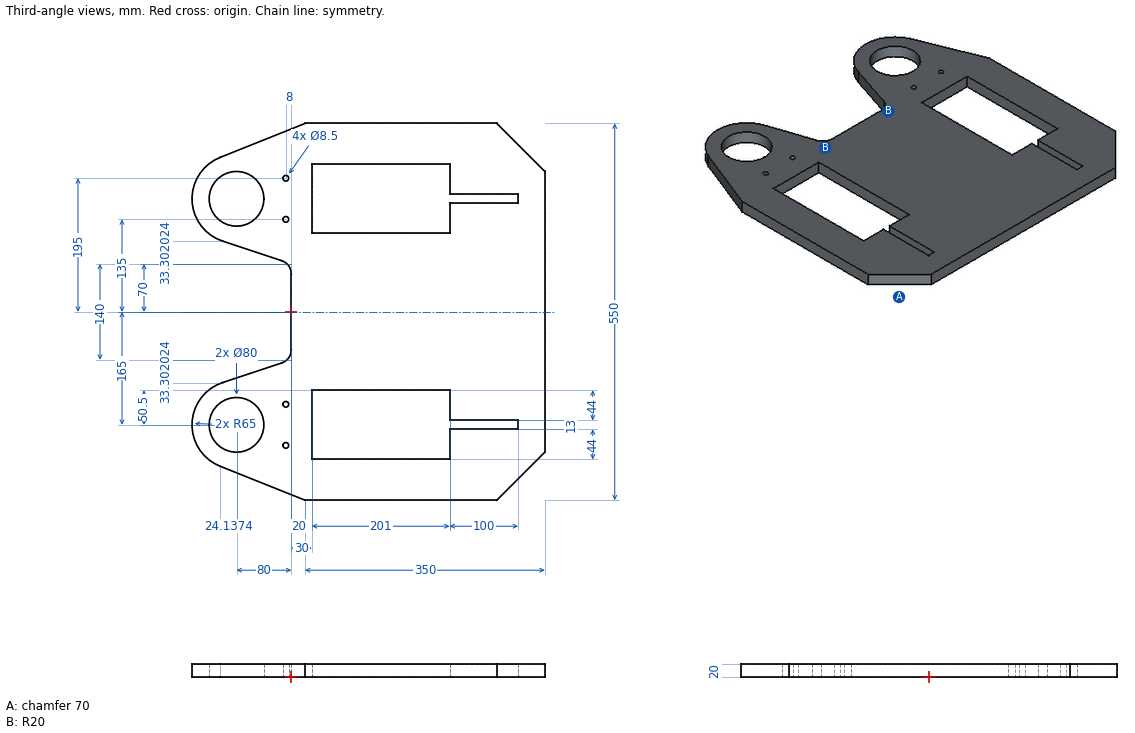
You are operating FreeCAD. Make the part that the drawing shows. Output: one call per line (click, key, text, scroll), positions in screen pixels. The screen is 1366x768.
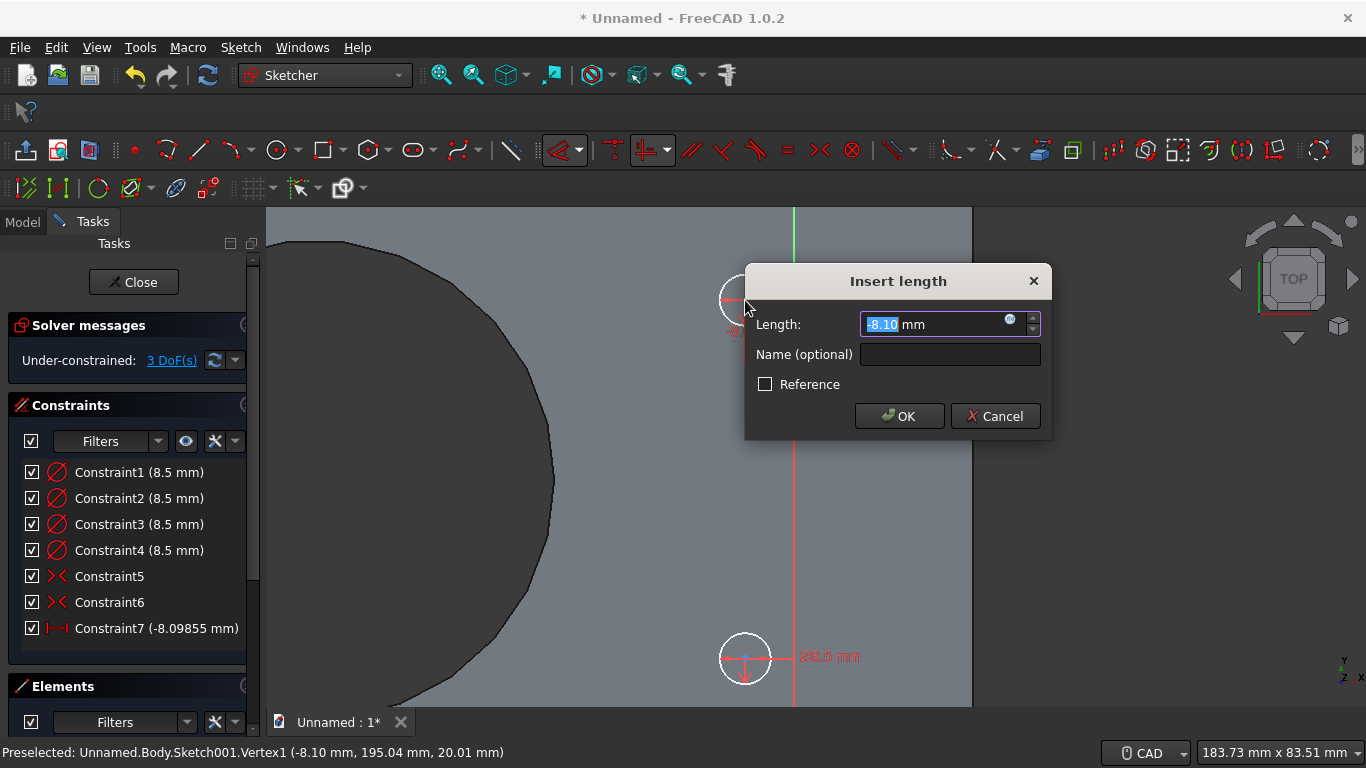
text(-8)
key(Return)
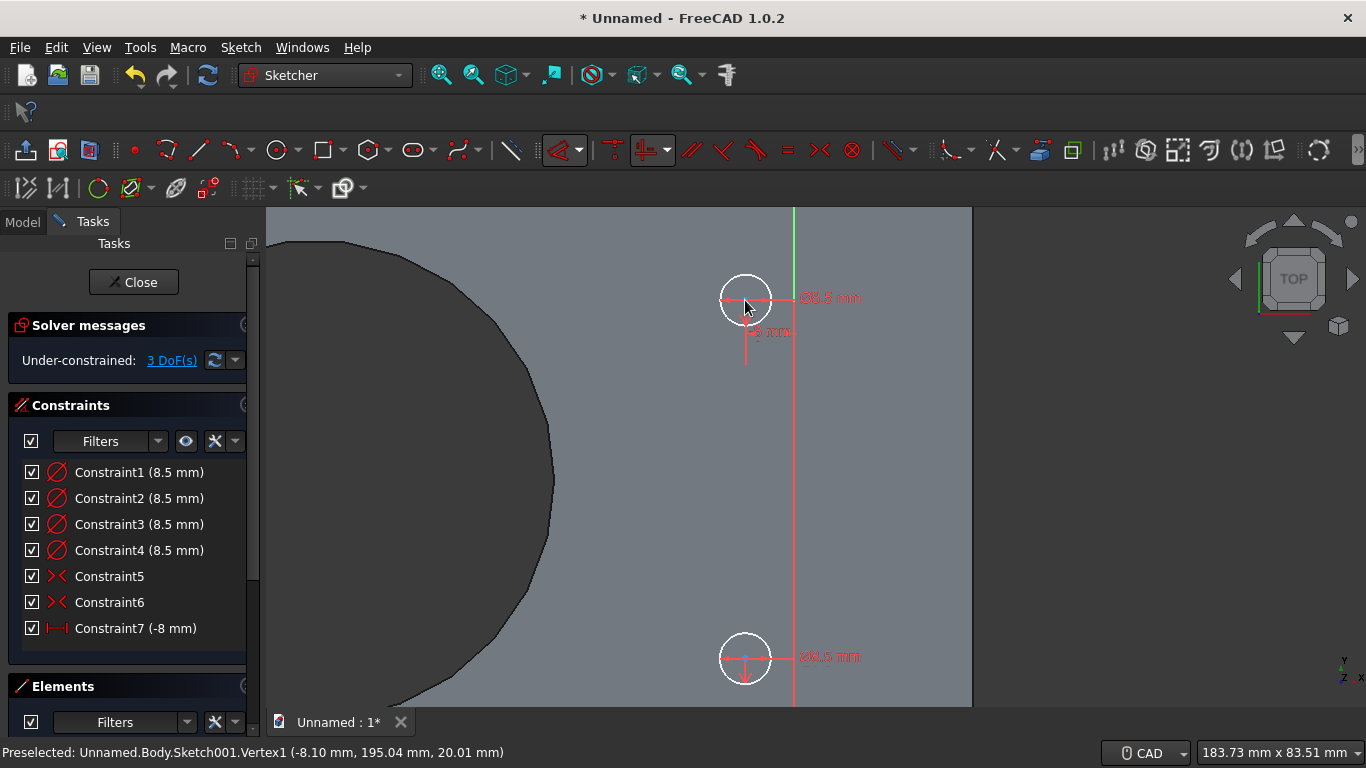
click(745, 659)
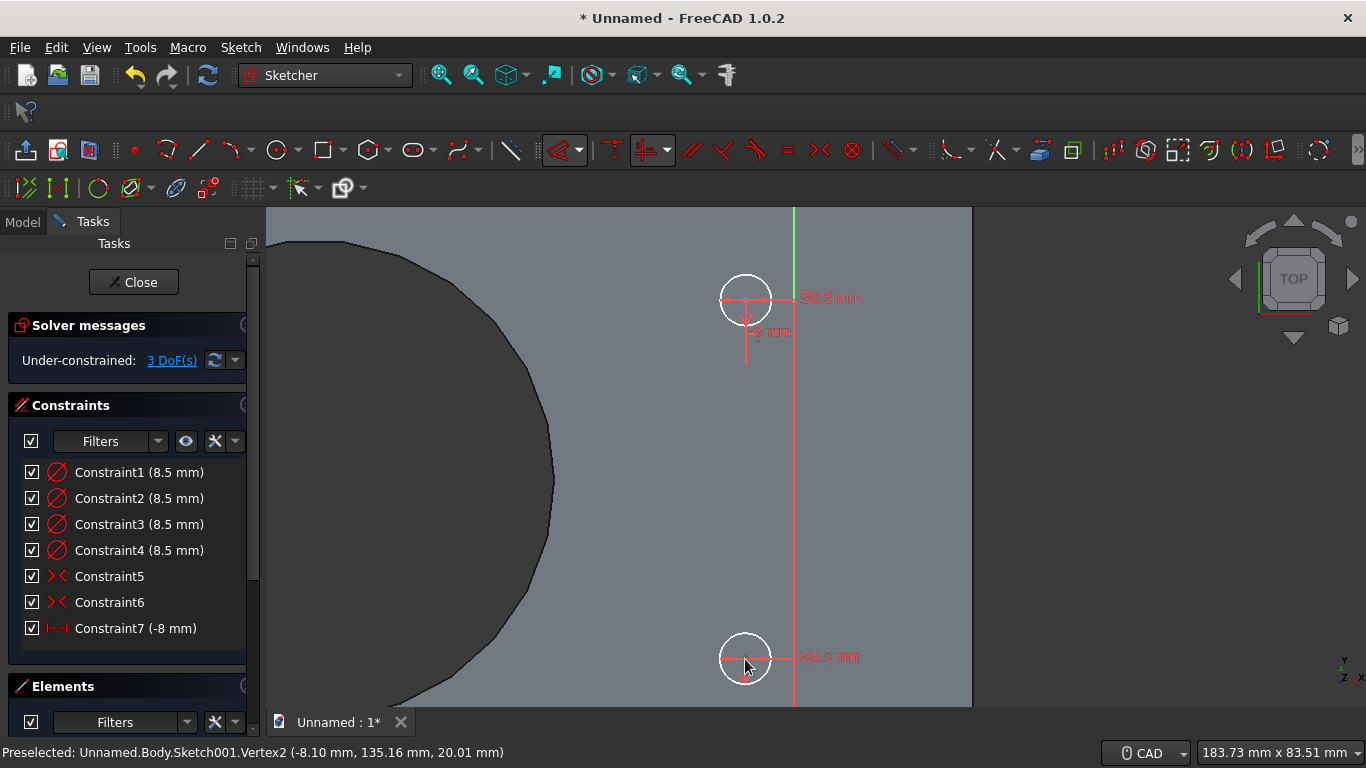
key(l)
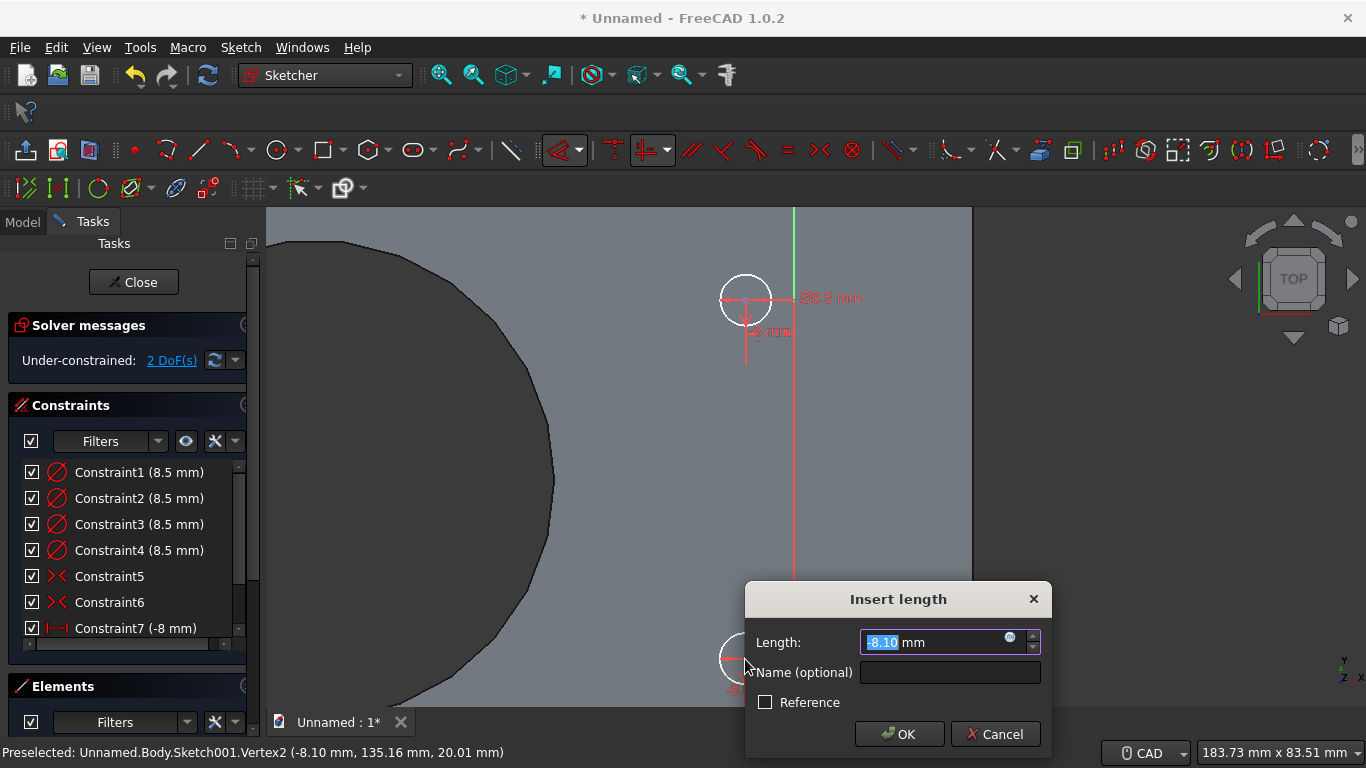
text(-8)
key(Return)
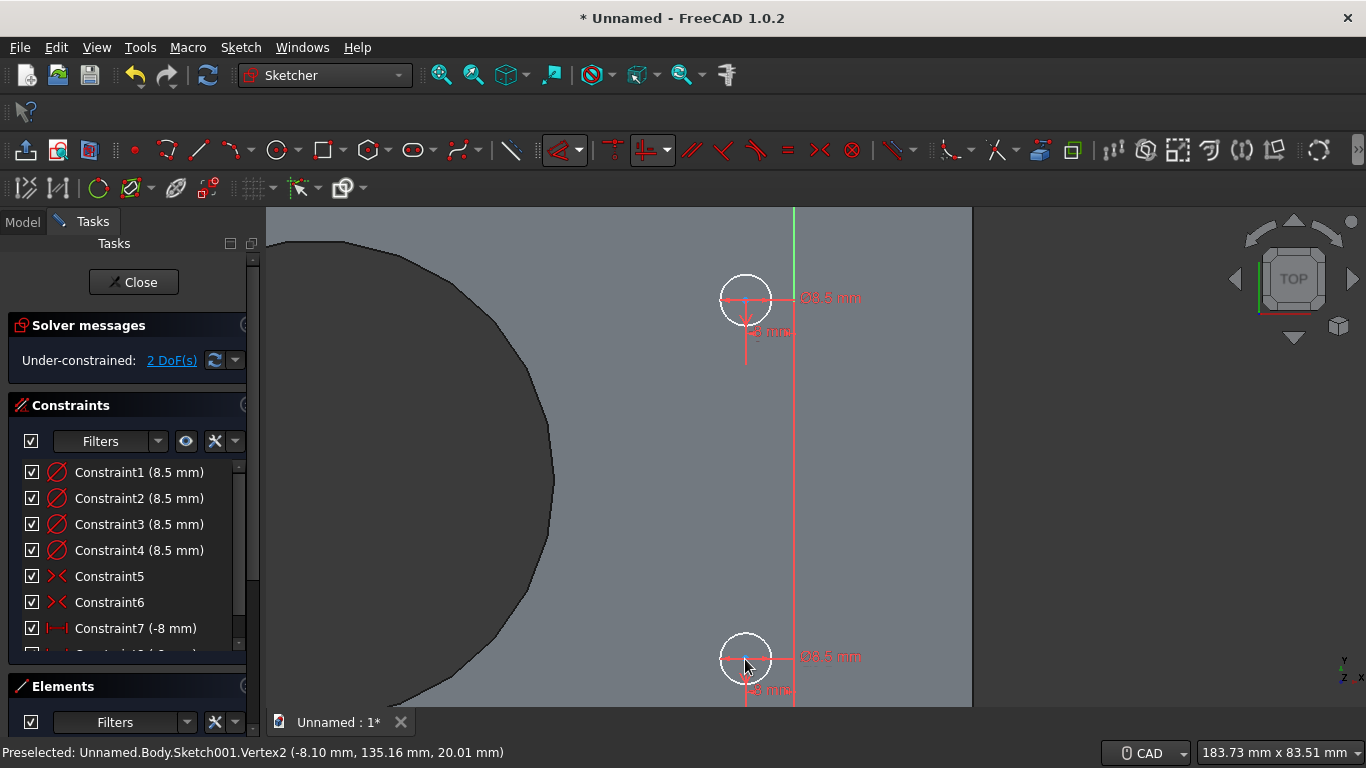
scroll(746, 299, down, 10)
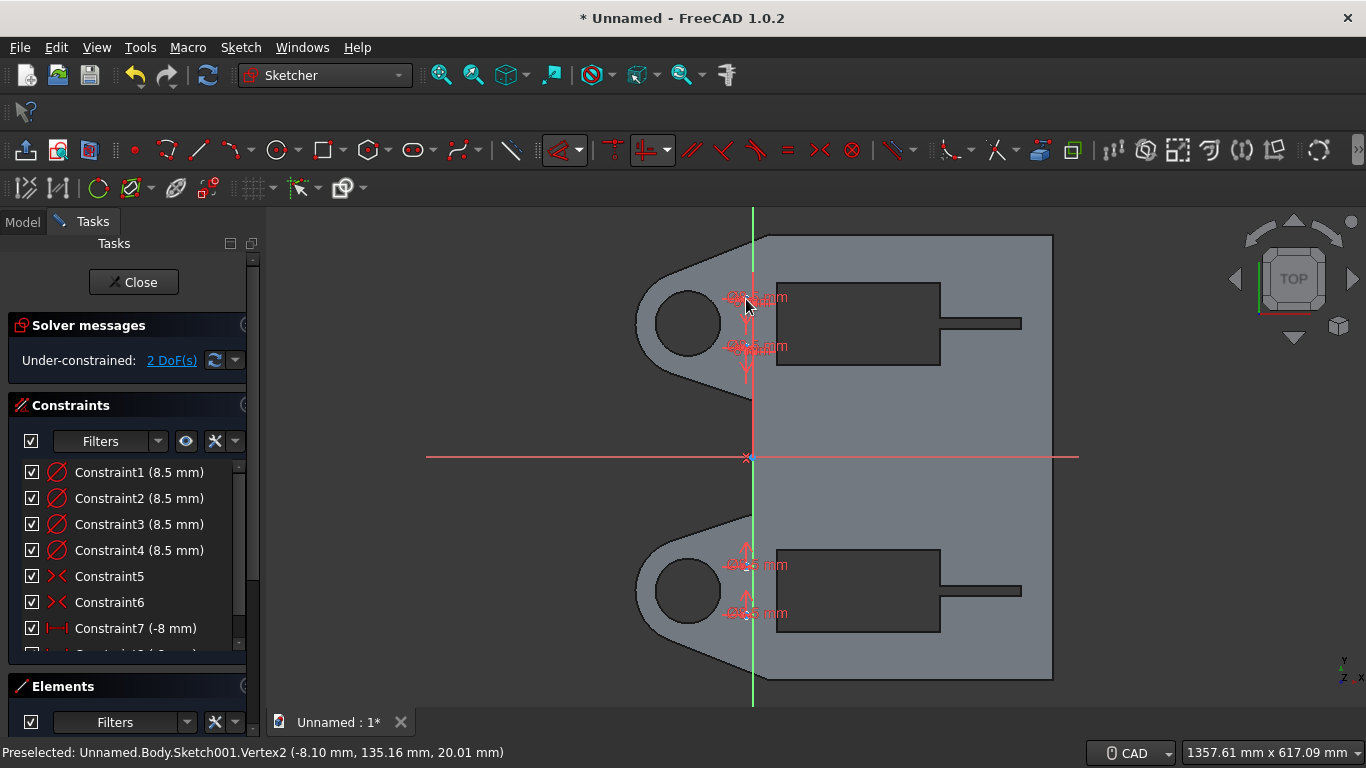
click(746, 299)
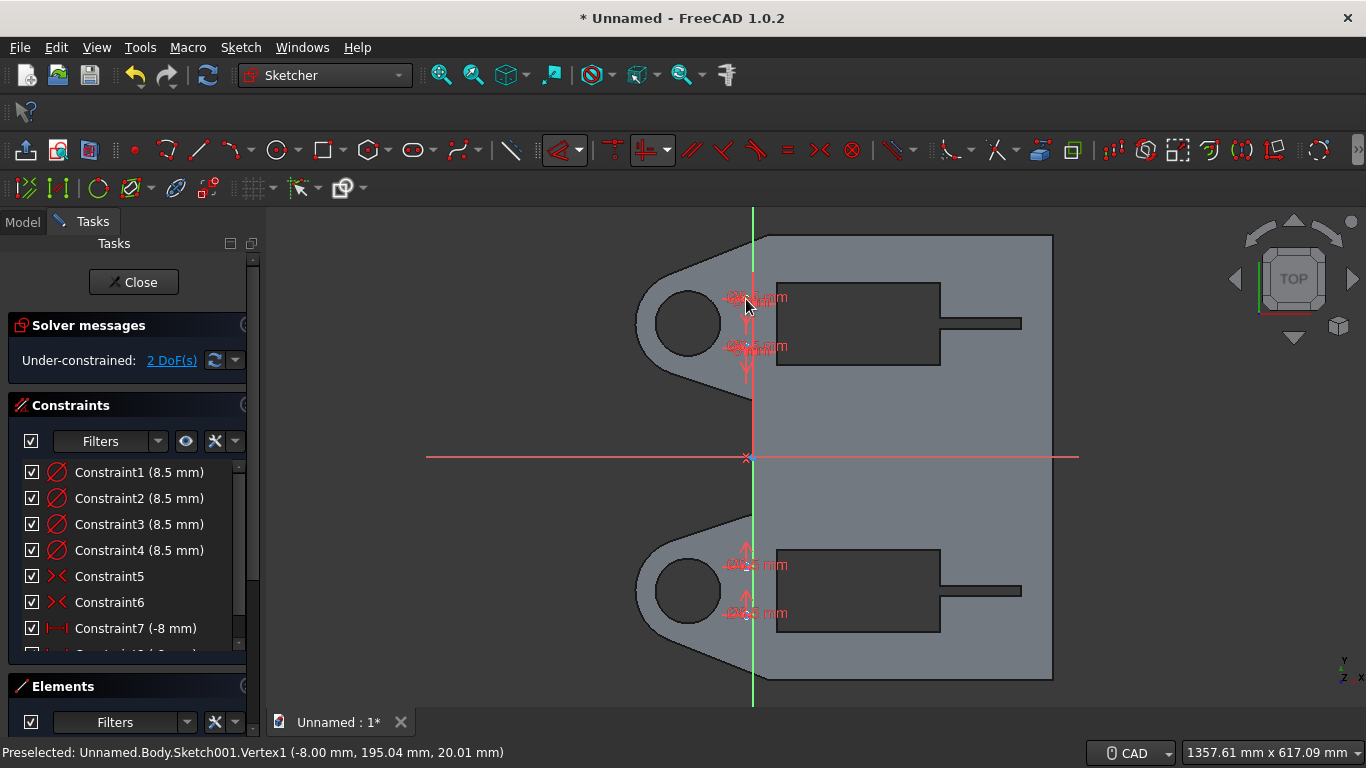
click(582, 150)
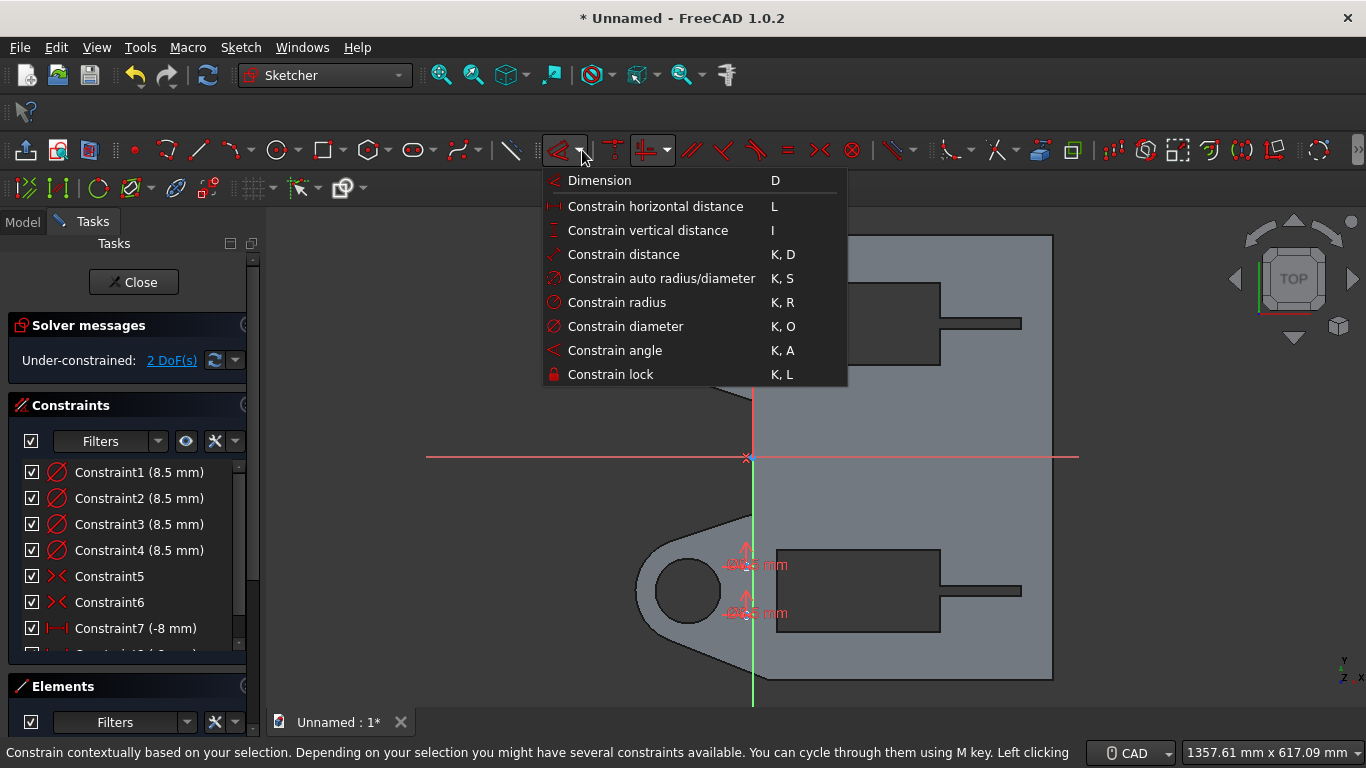
click(695, 230)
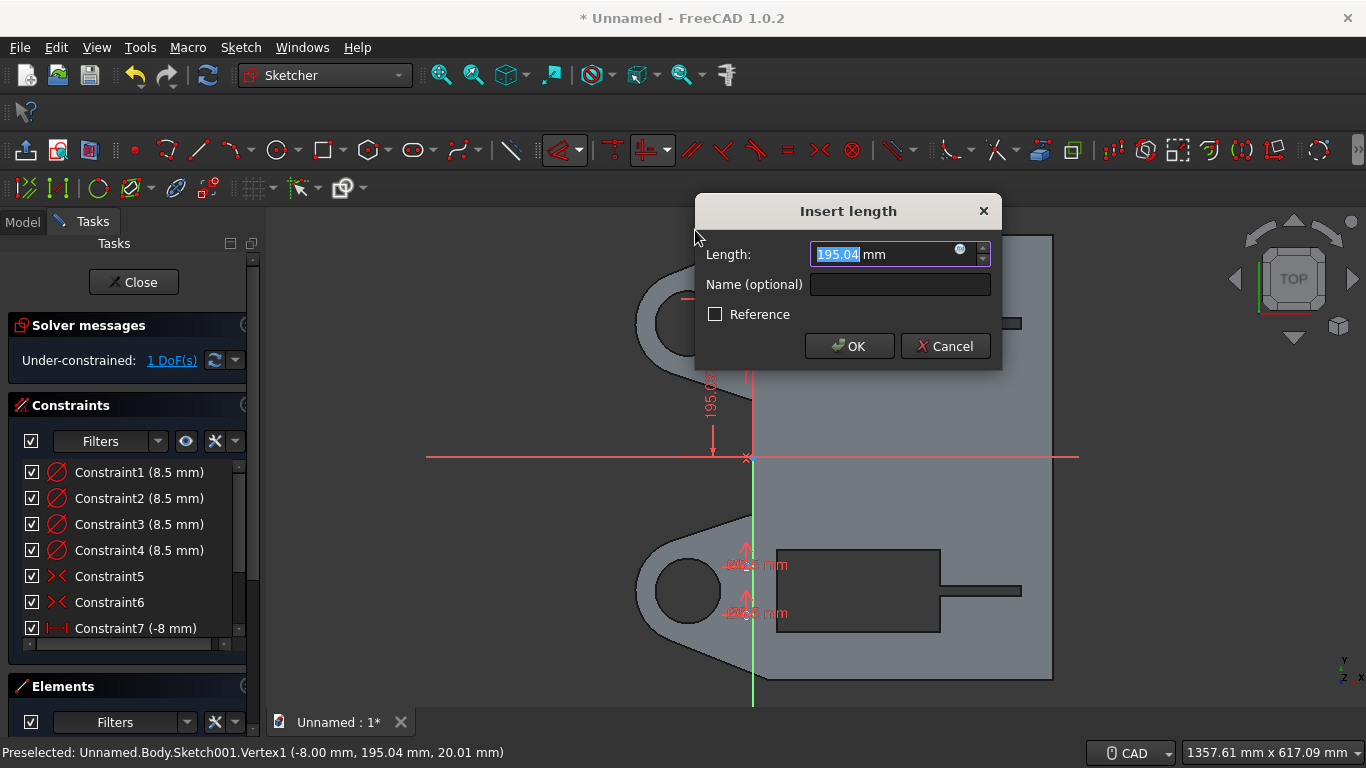
text(195)
key(Return)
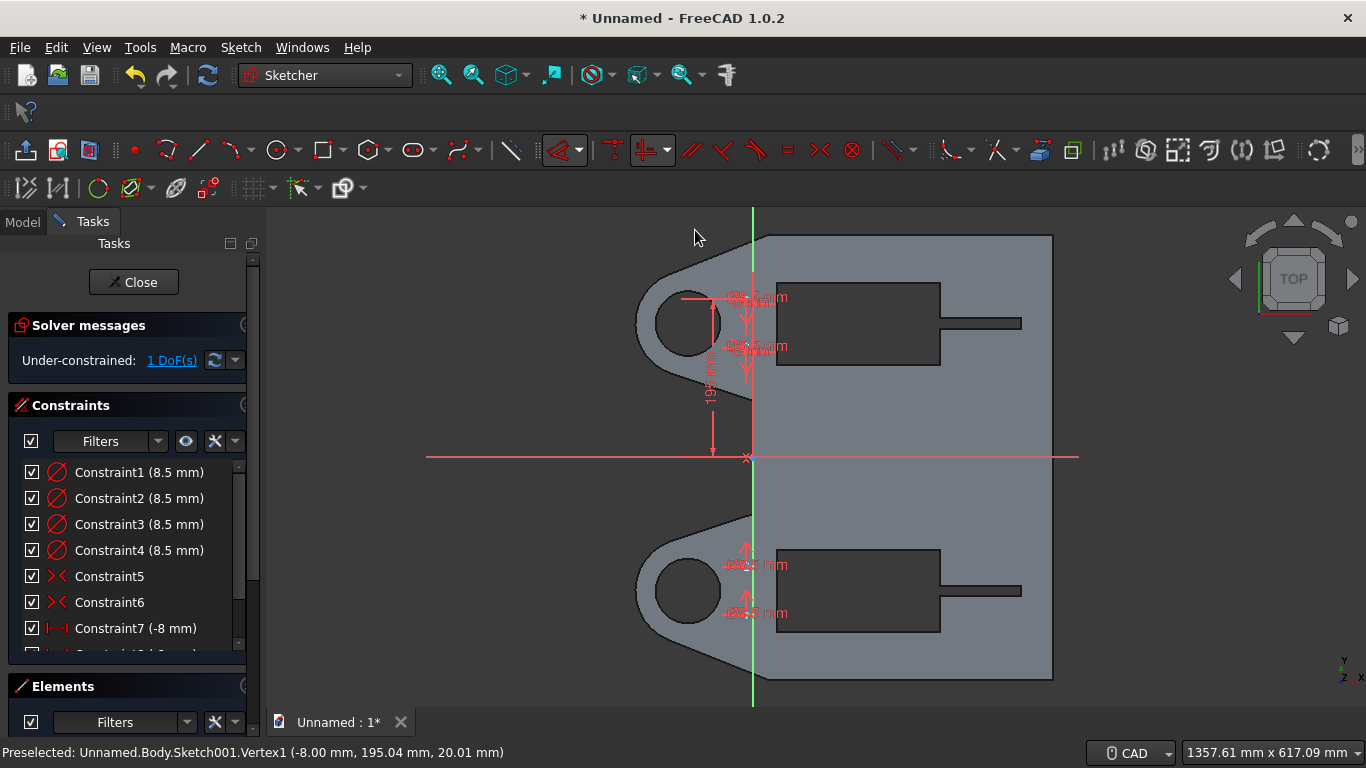
click(746, 348)